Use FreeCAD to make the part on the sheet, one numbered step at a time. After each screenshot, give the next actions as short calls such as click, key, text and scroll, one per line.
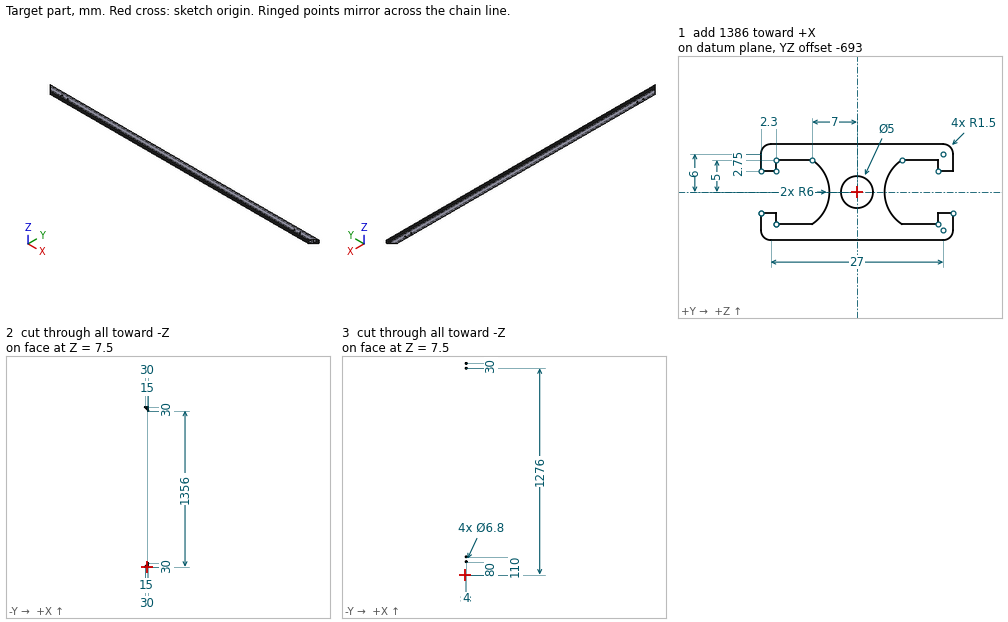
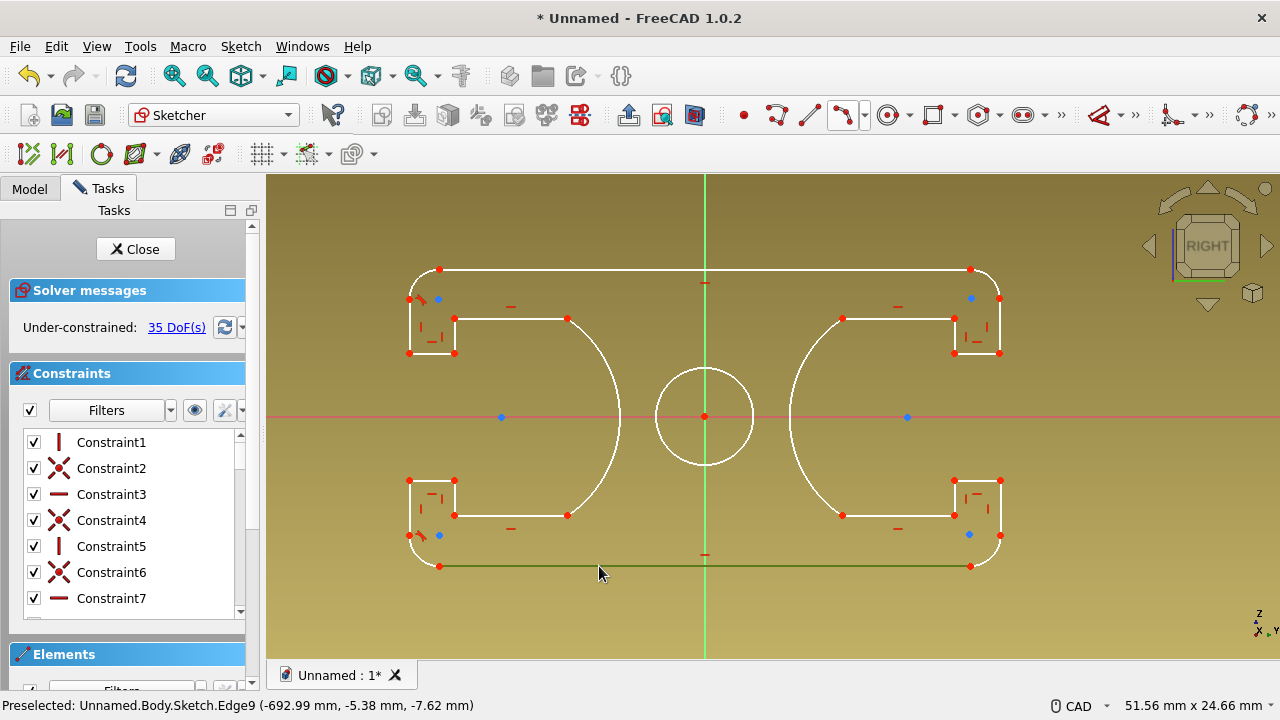
click(413, 550)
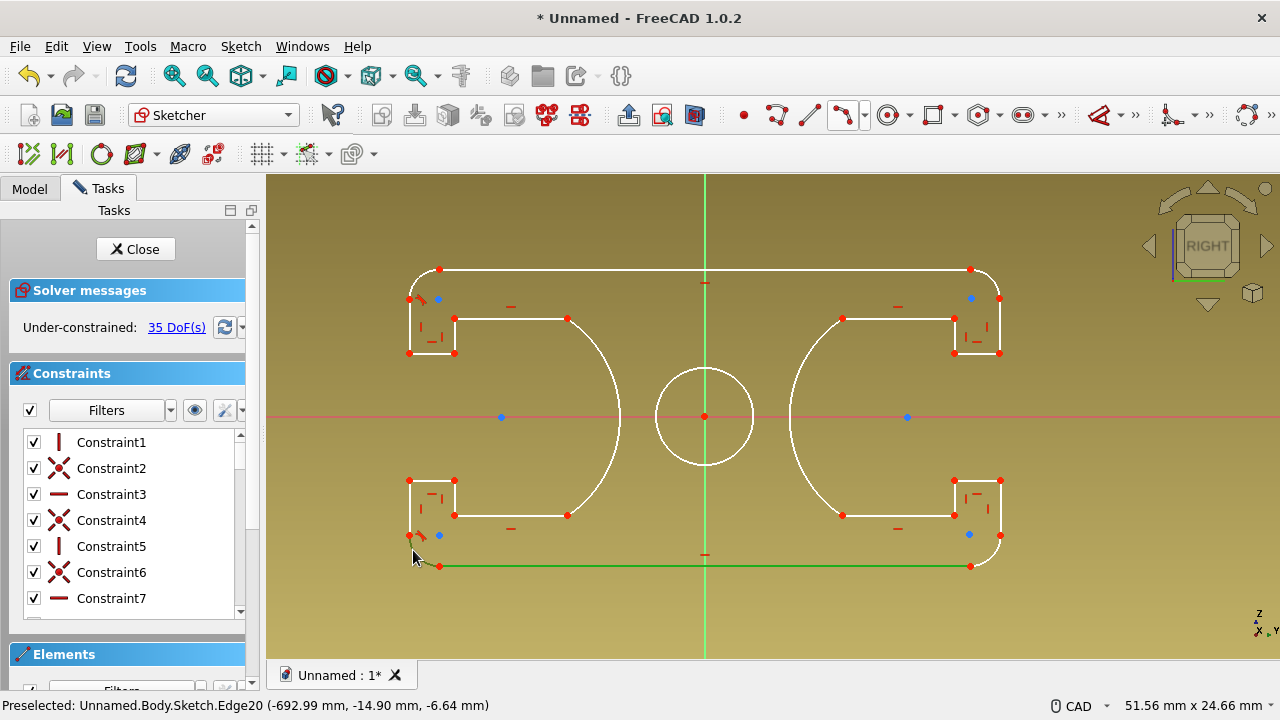
key(t)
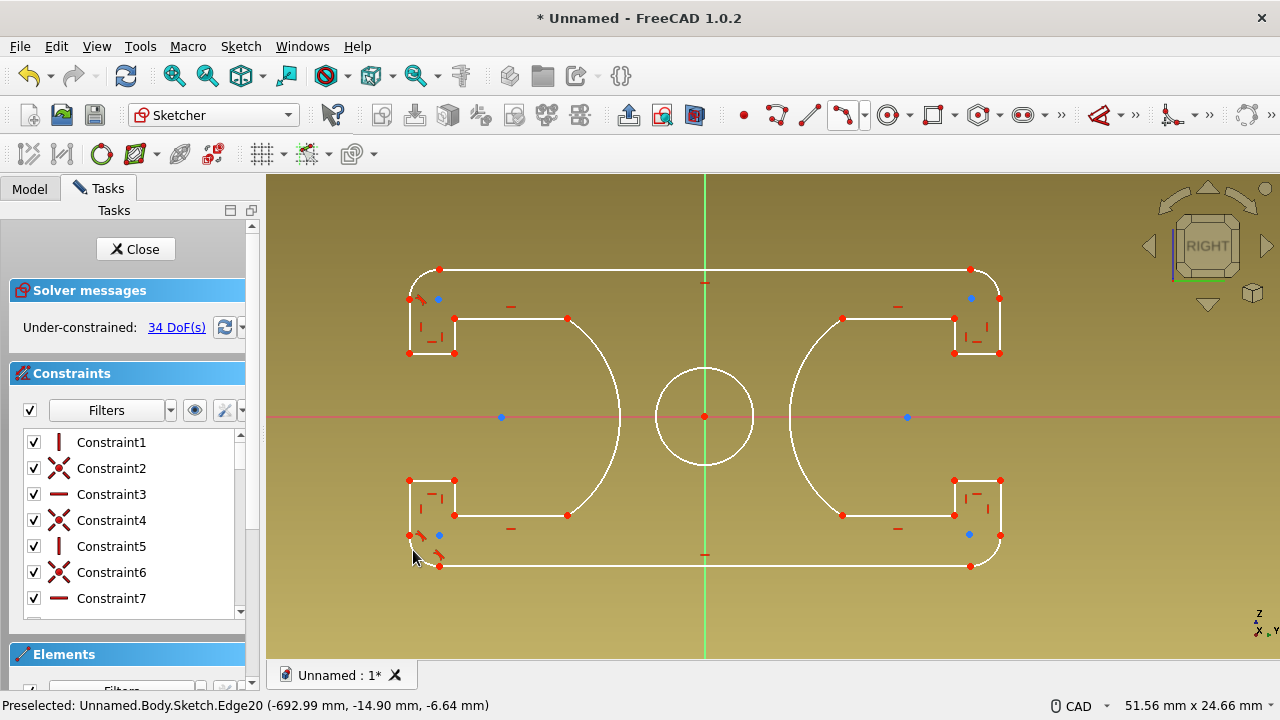
click(599, 566)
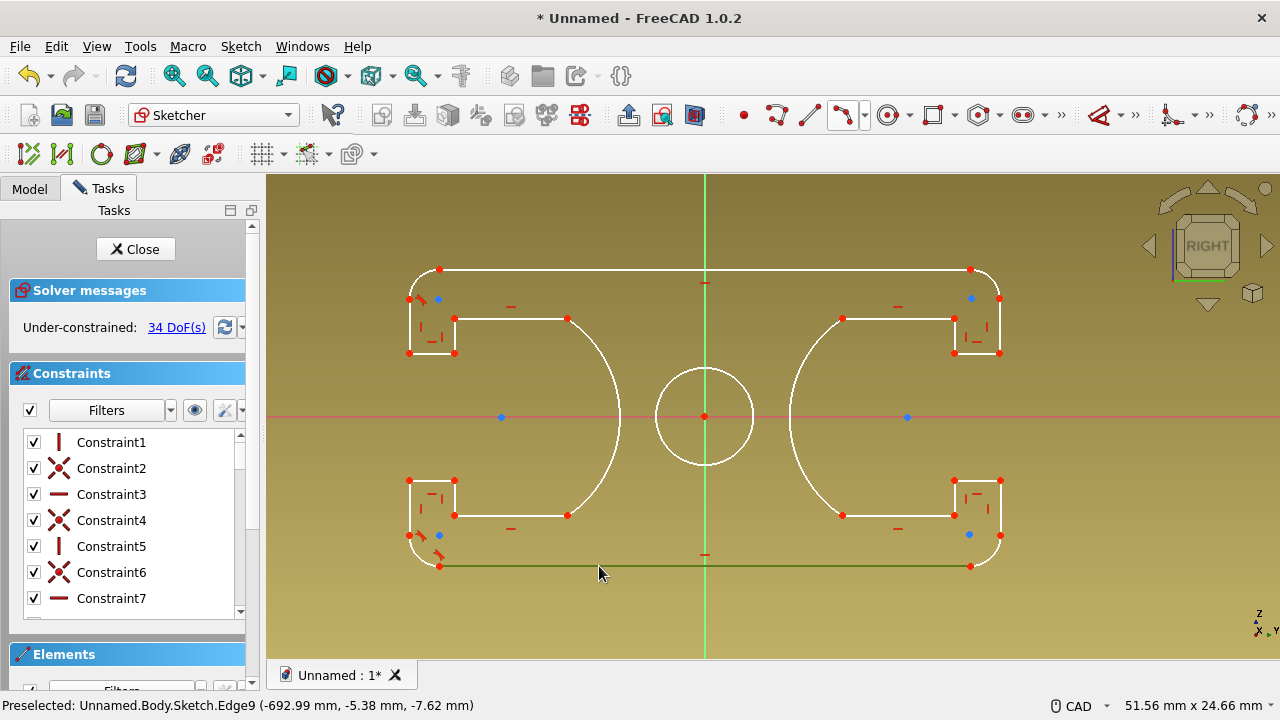
click(984, 563)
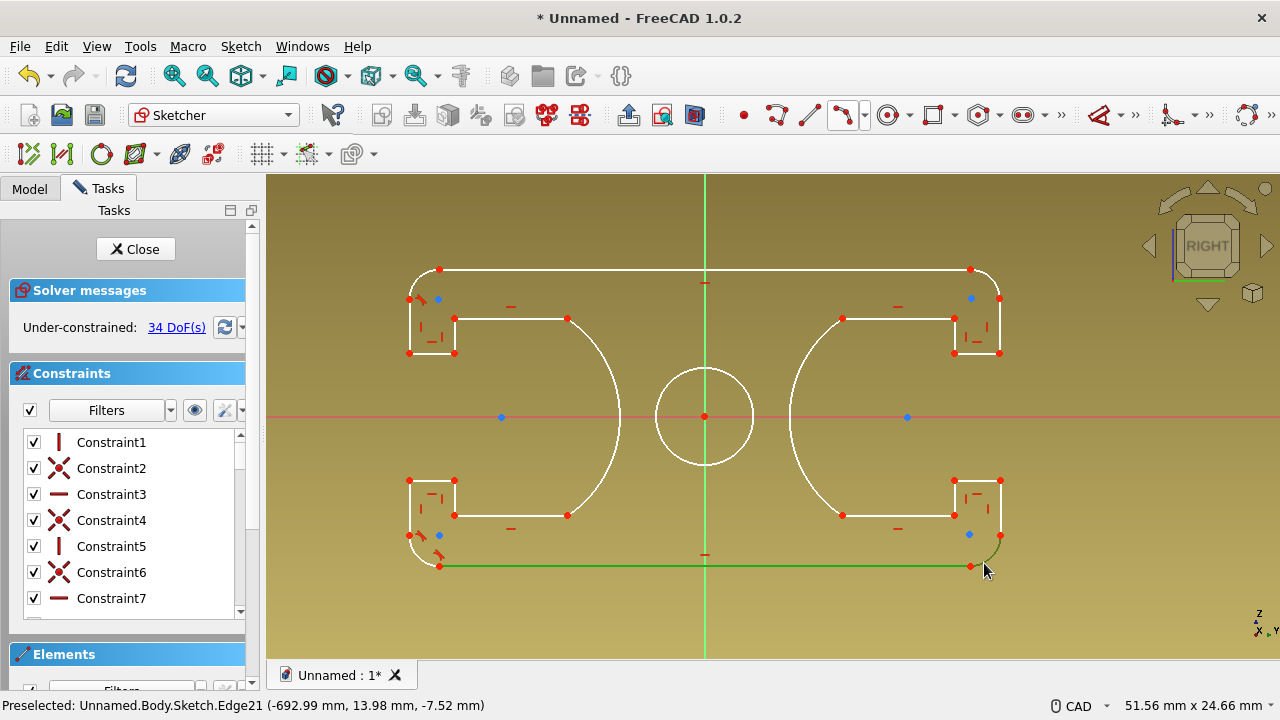
key(t)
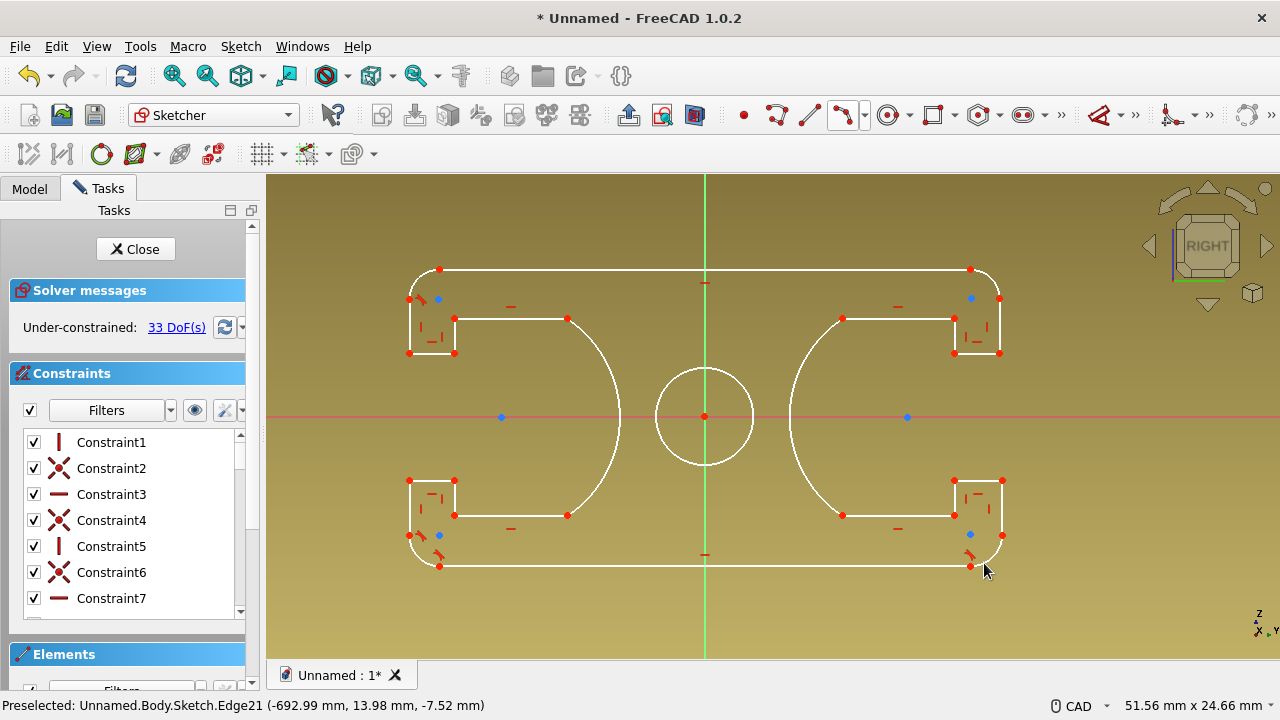
click(1002, 519)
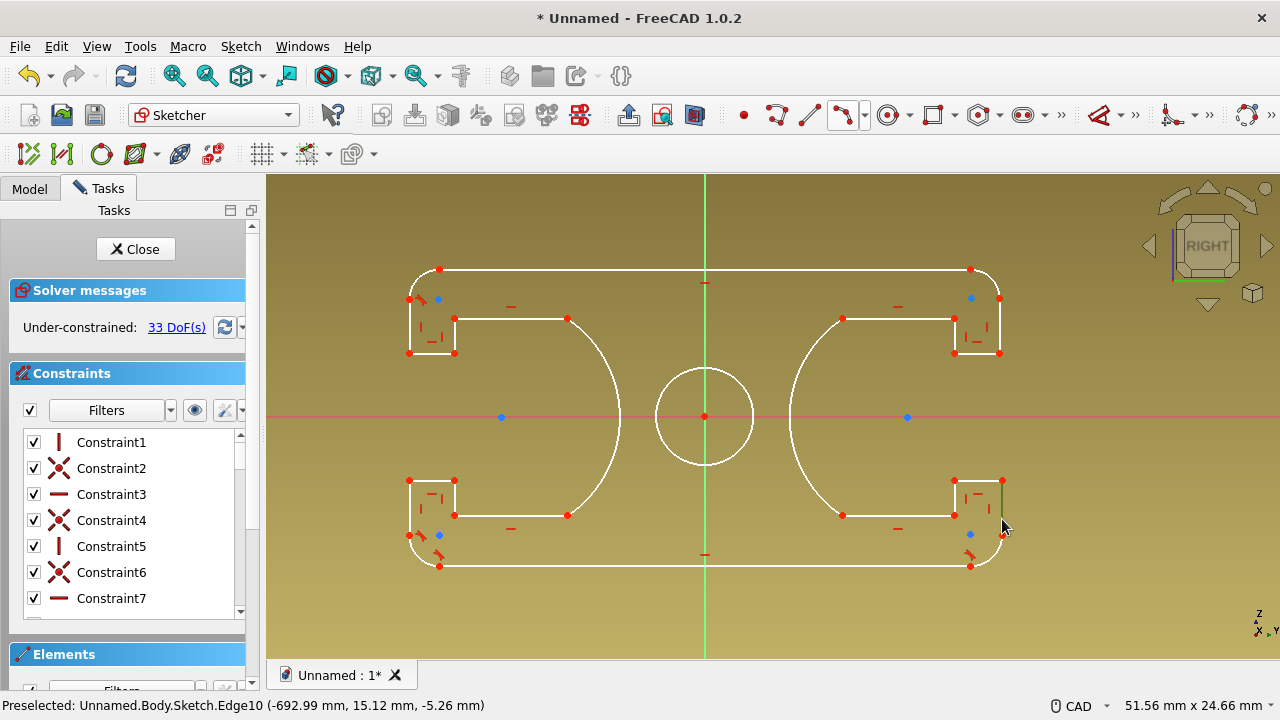
click(985, 563)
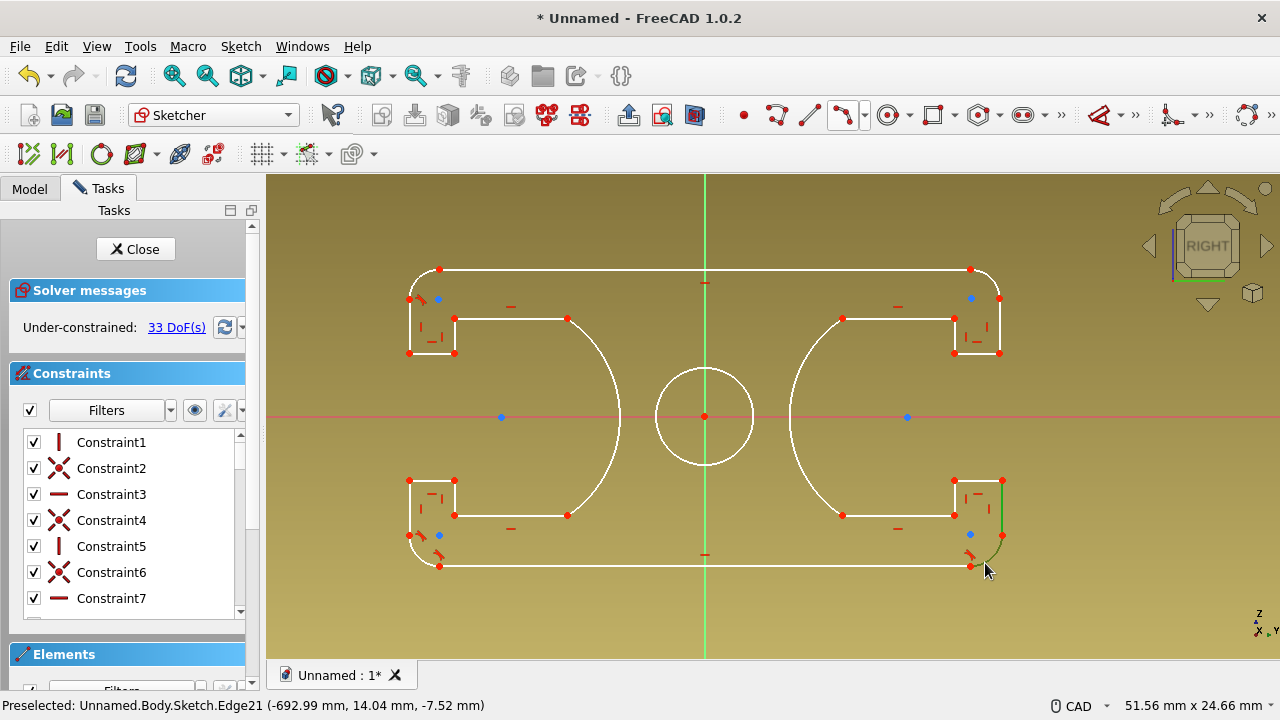
key(t)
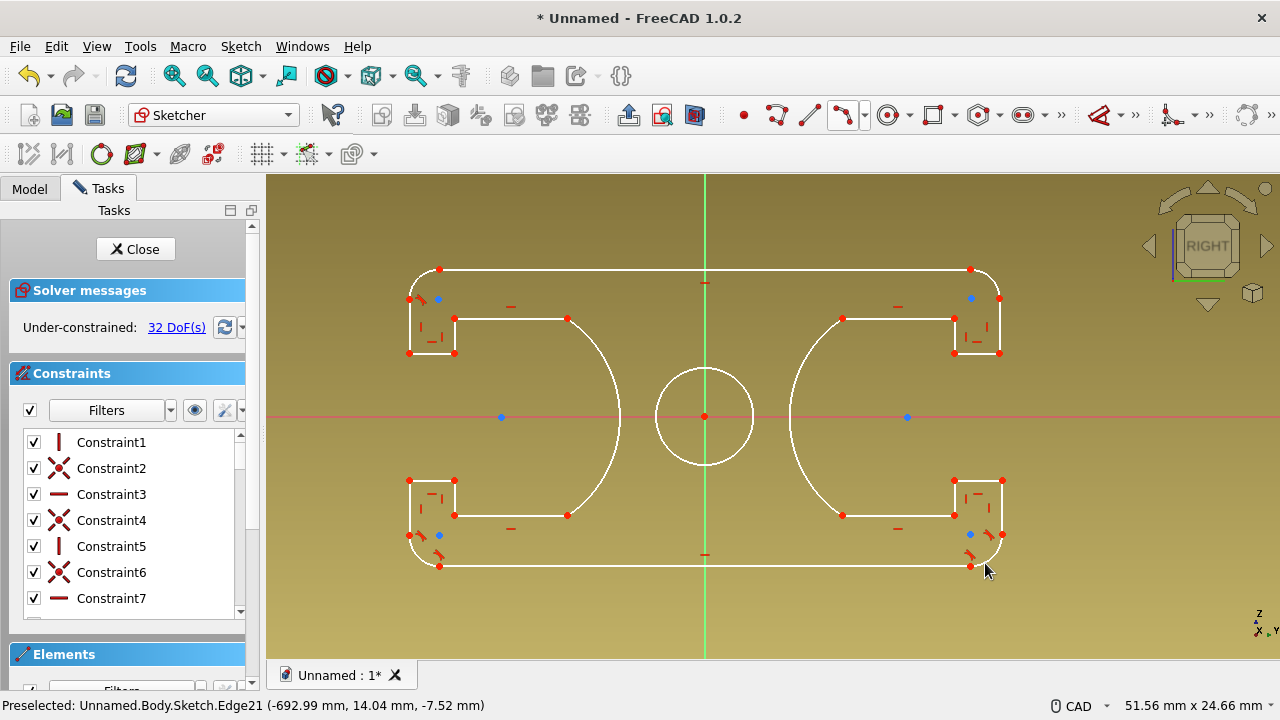
click(1000, 337)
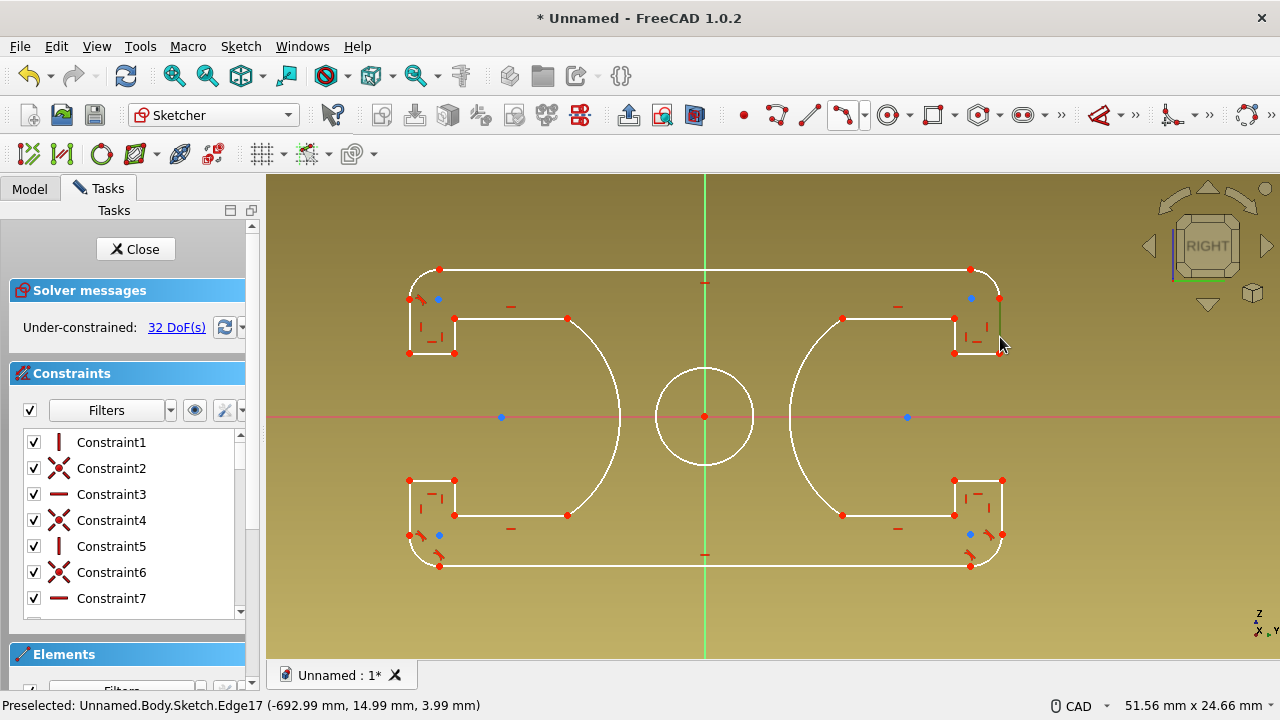
click(997, 286)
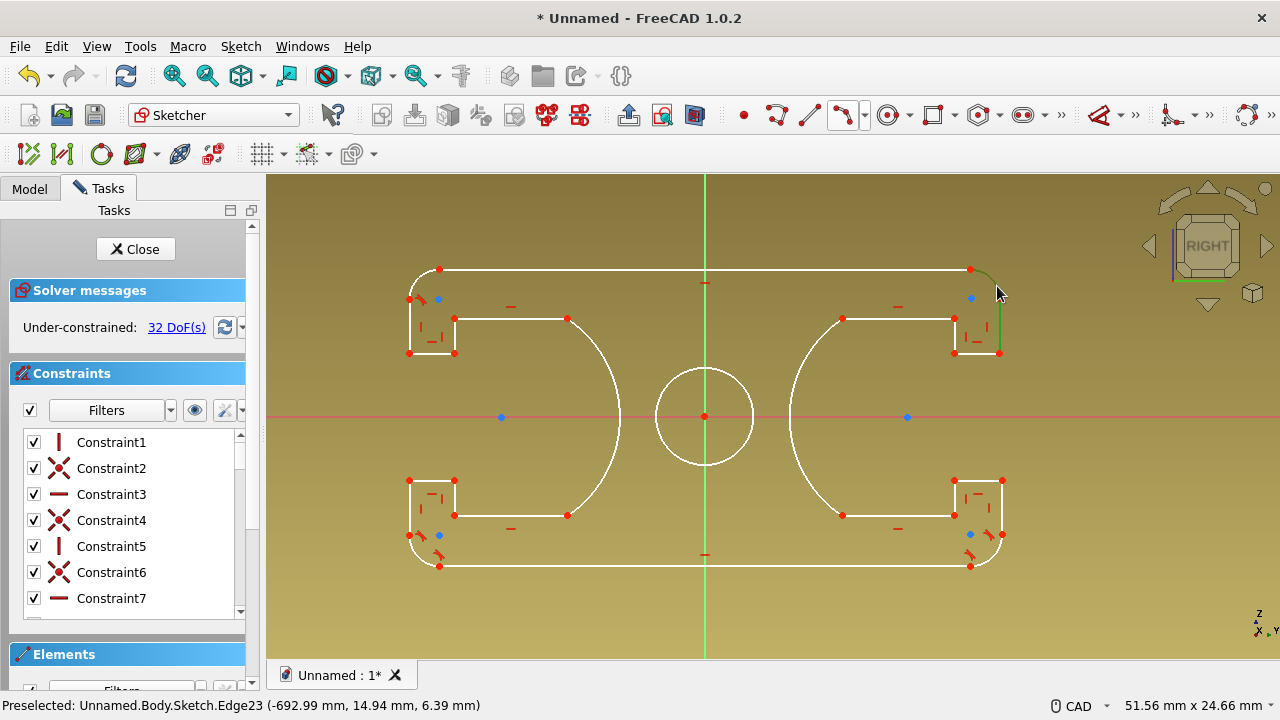
key(t)